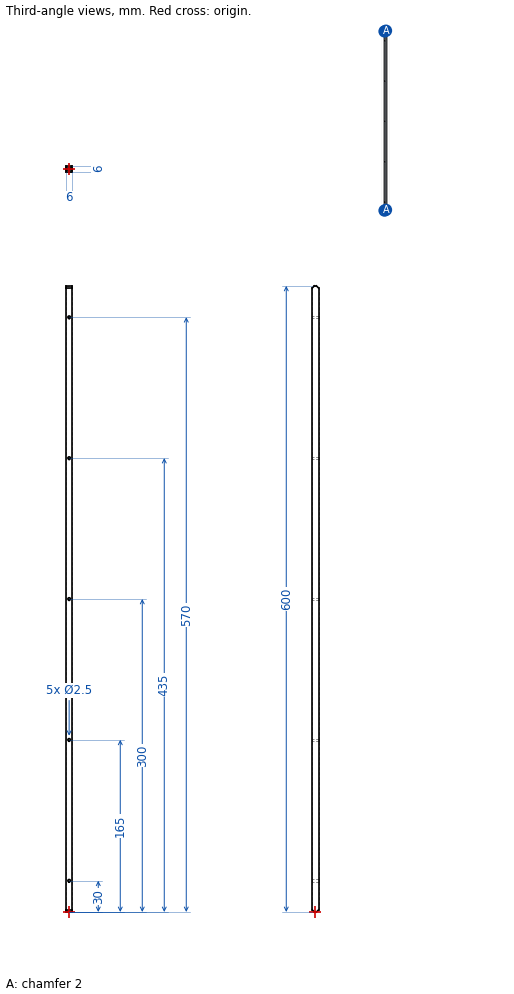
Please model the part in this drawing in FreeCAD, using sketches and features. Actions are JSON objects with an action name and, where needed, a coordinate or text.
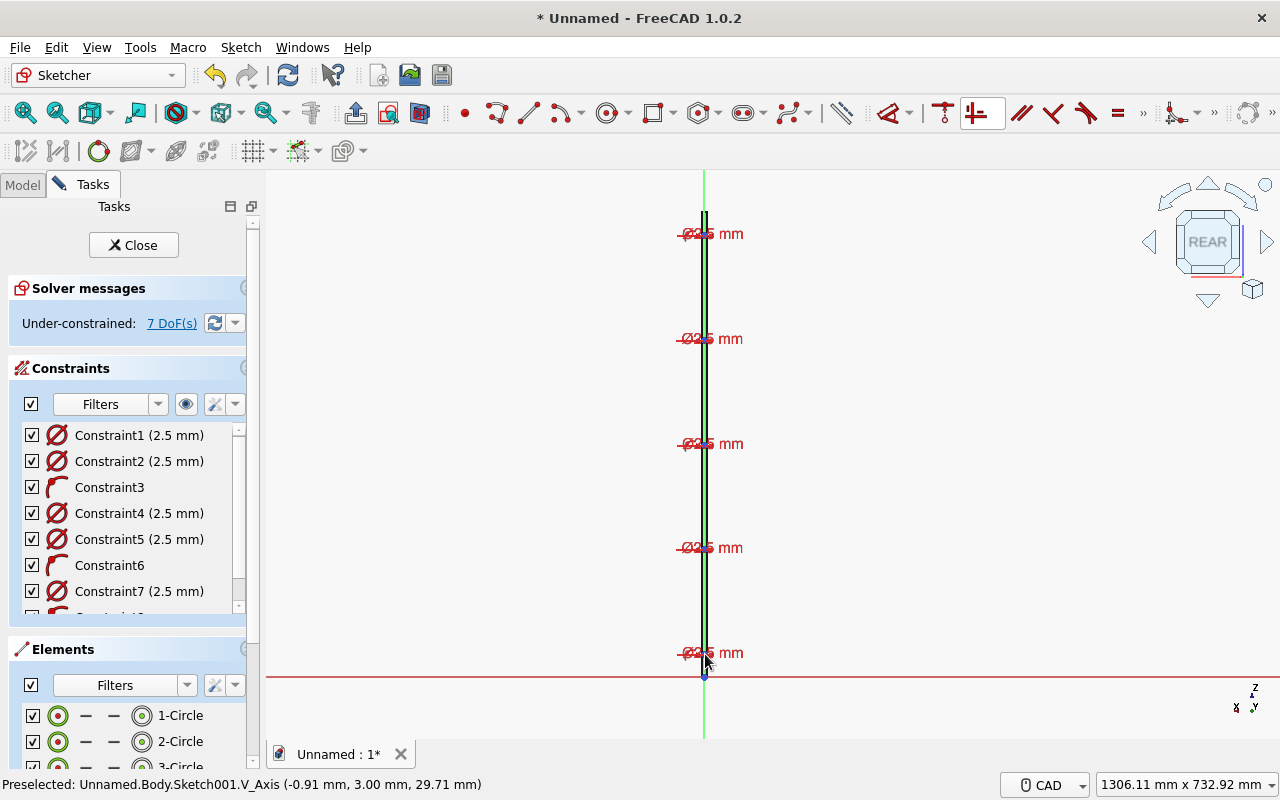
{"action": "left_click", "coordinate": [704, 550]}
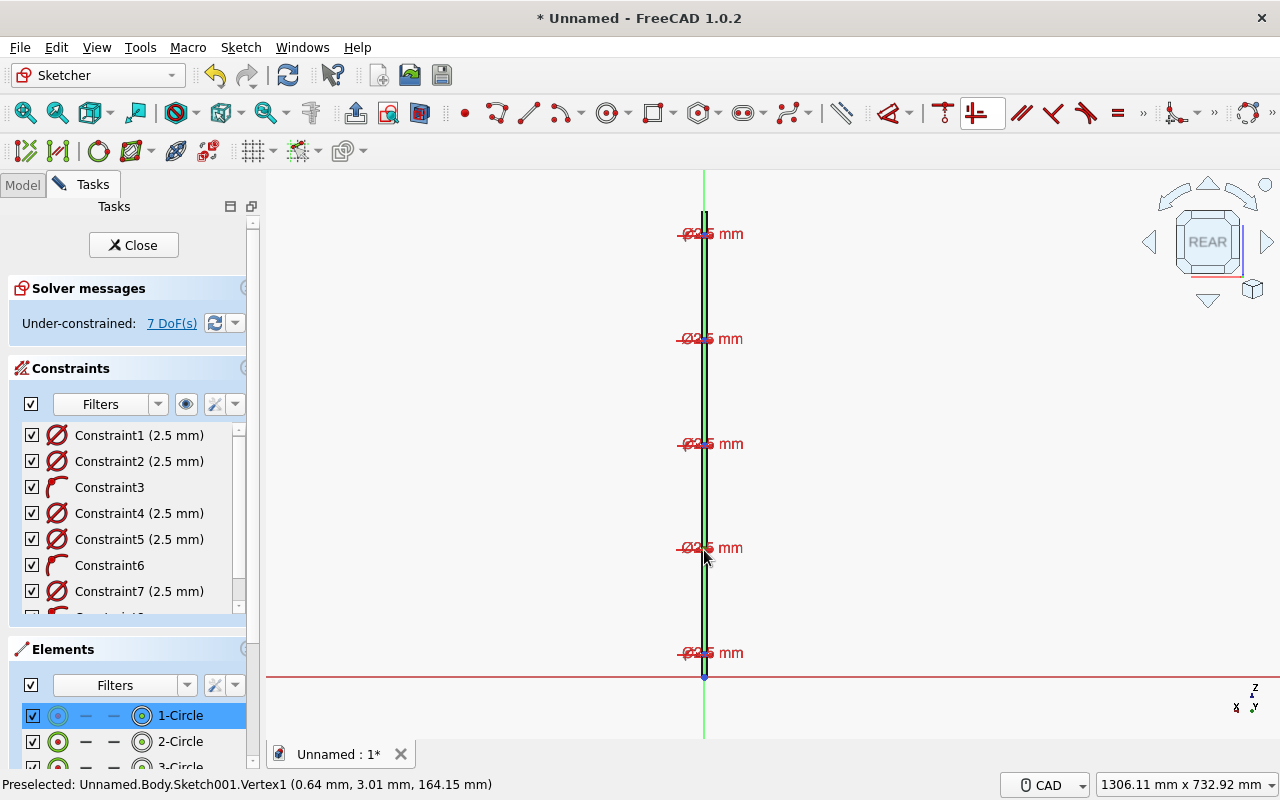
{"action": "left_click", "coordinate": [704, 601]}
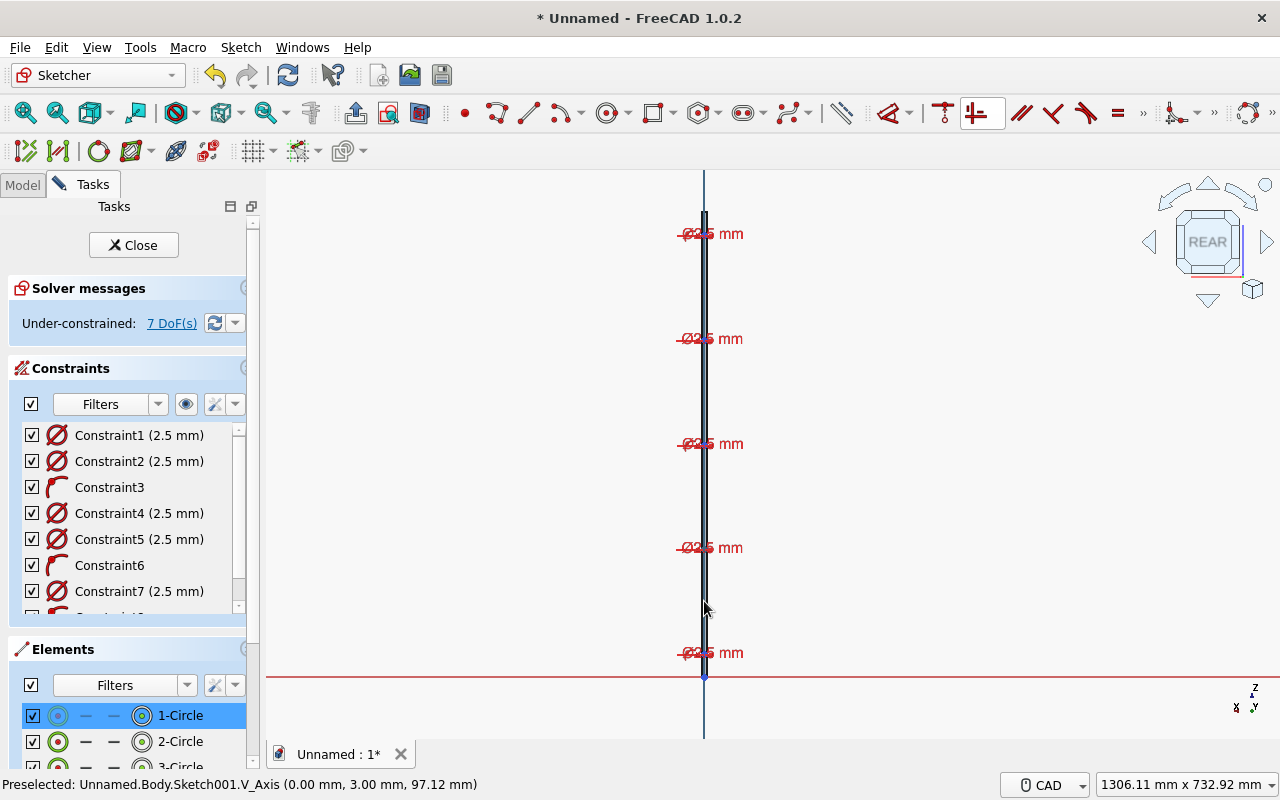
{"action": "left_click", "coordinate": [944, 114]}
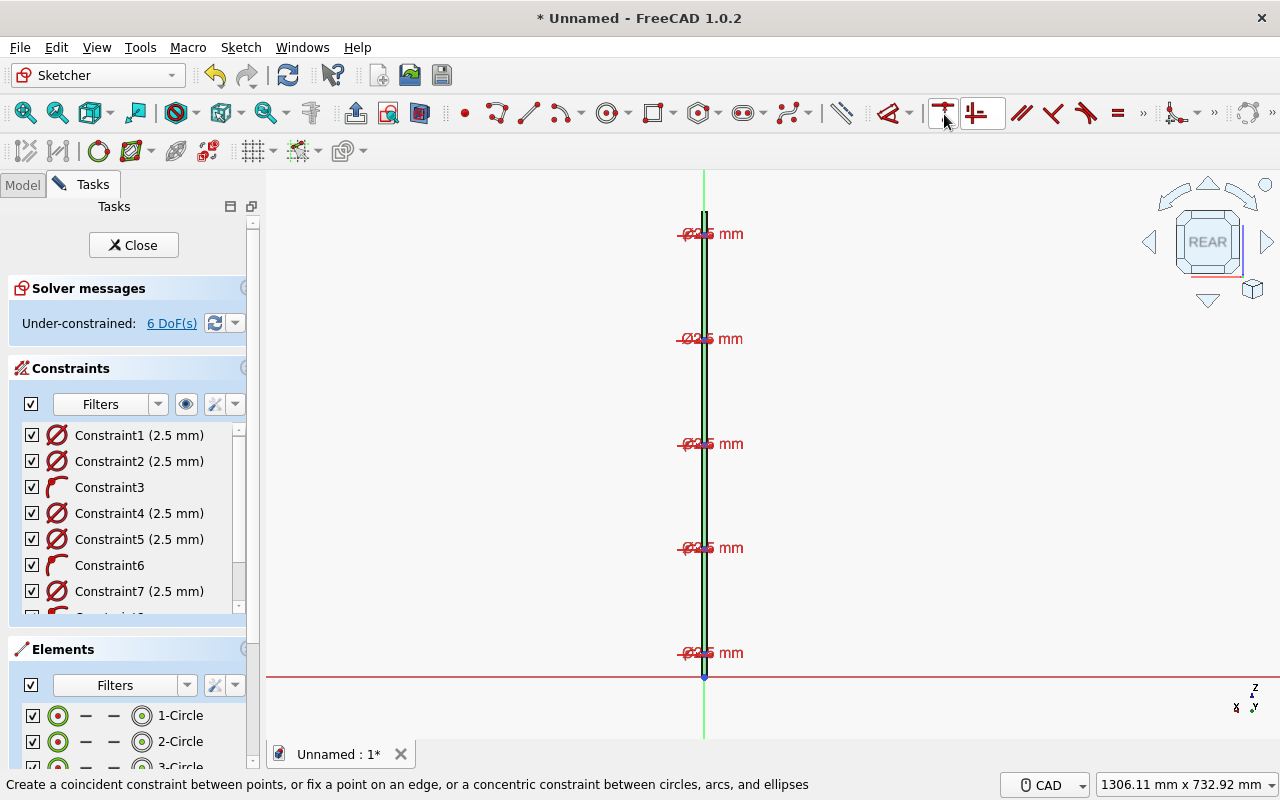
{"action": "left_click", "coordinate": [704, 341]}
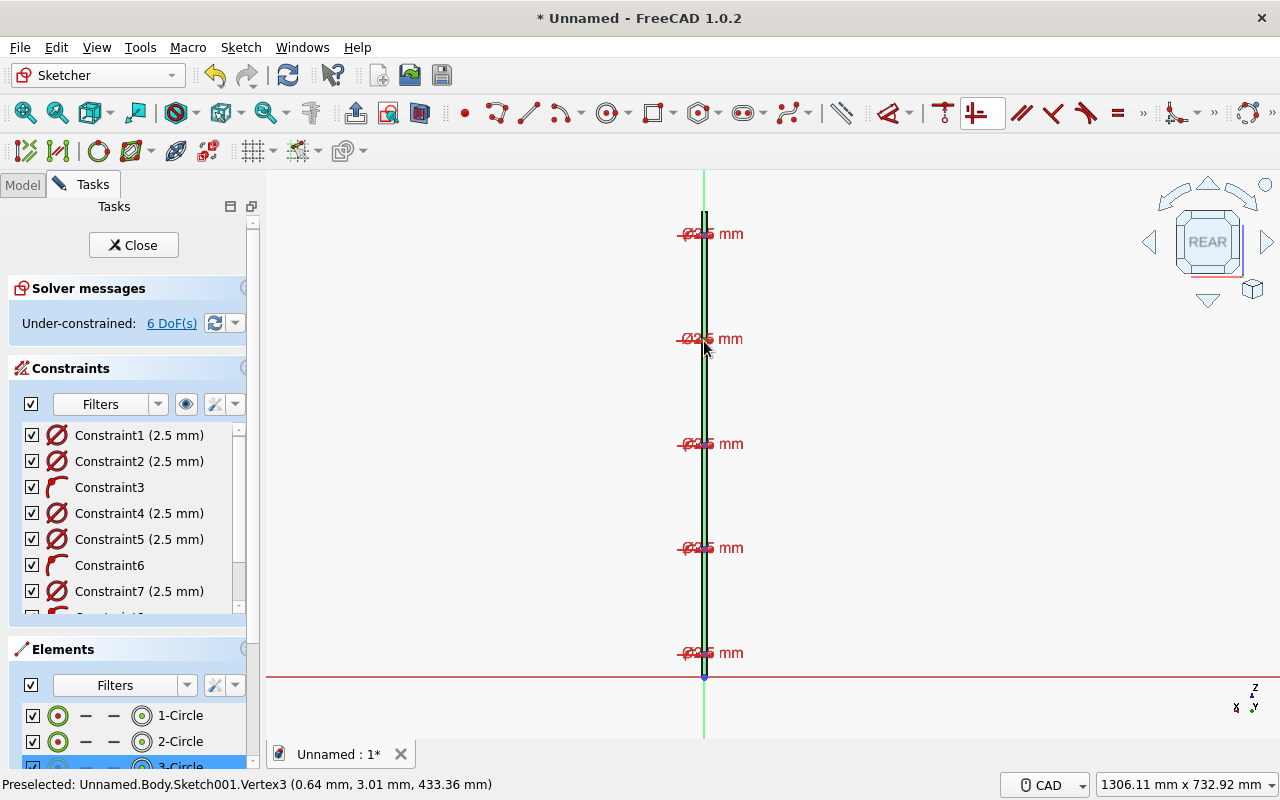
{"action": "left_click", "coordinate": [704, 601]}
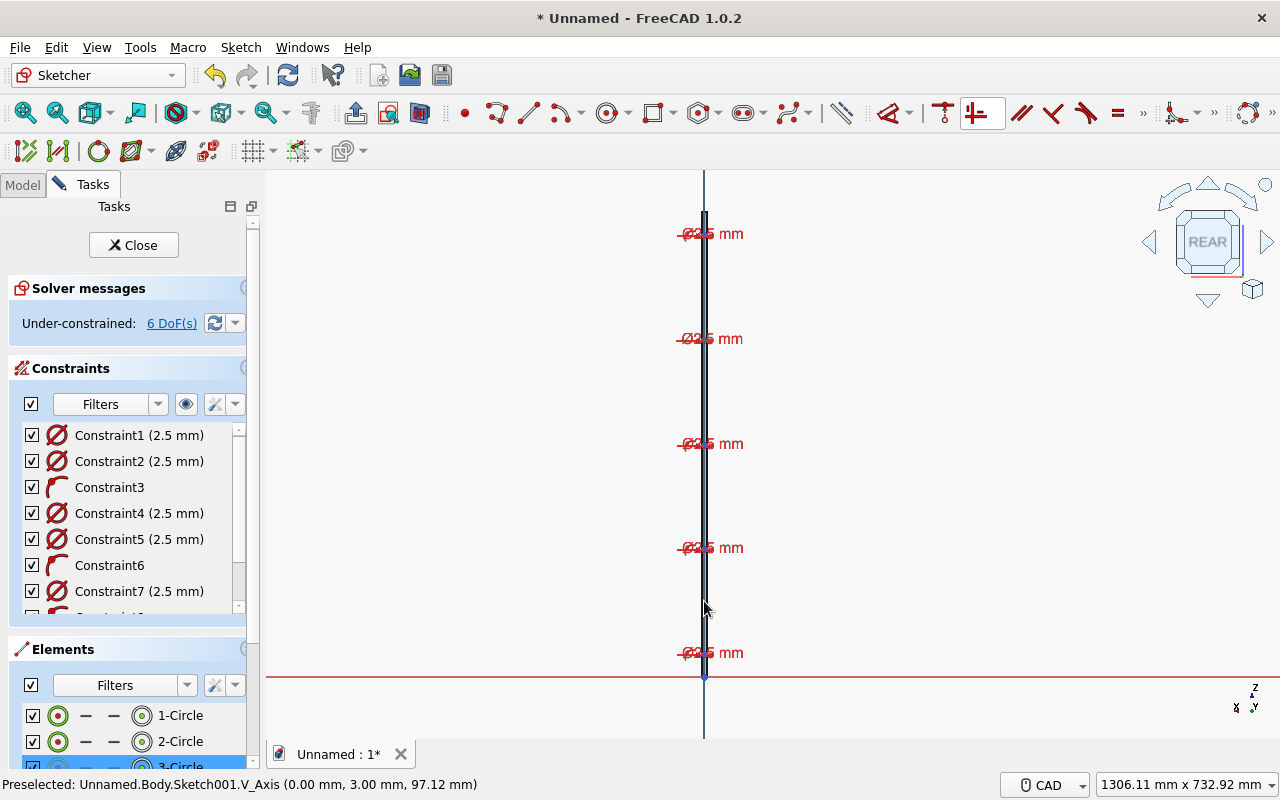
{"action": "left_click", "coordinate": [944, 114]}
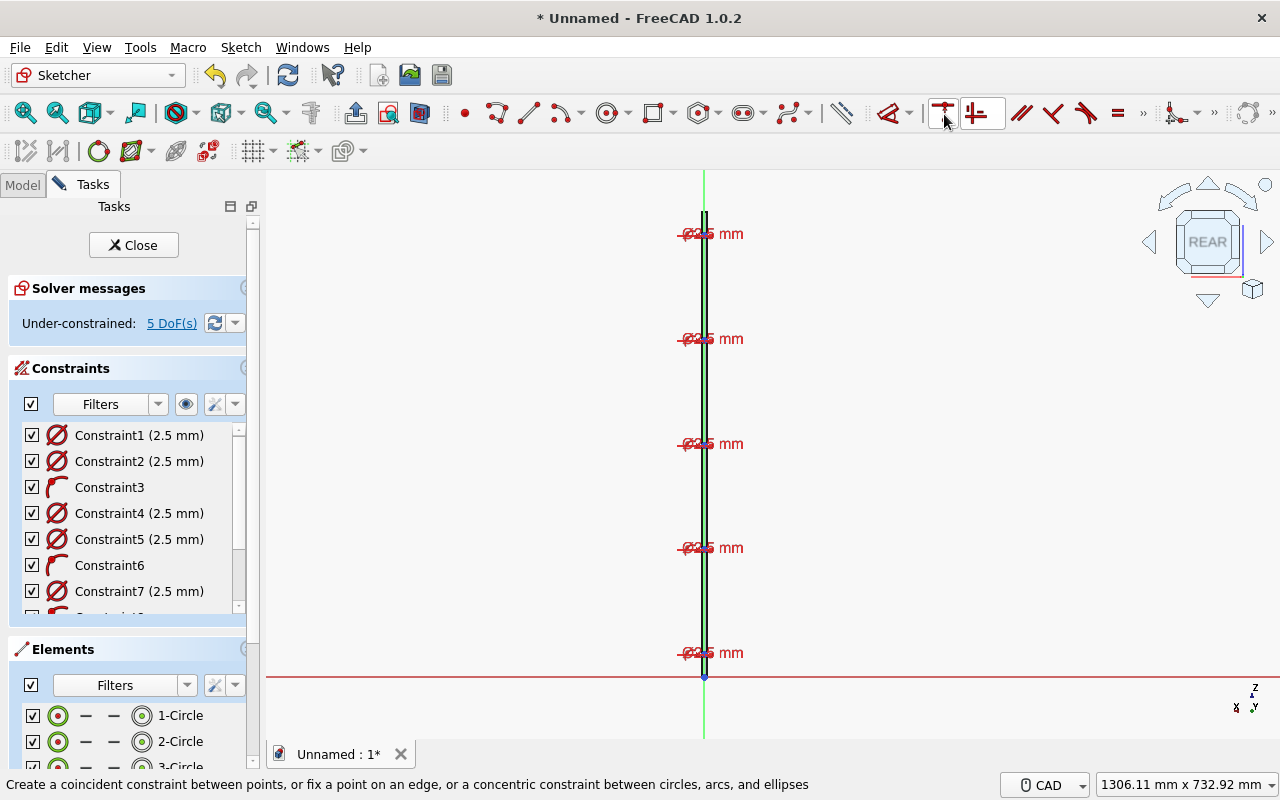
{"action": "left_click", "coordinate": [888, 114]}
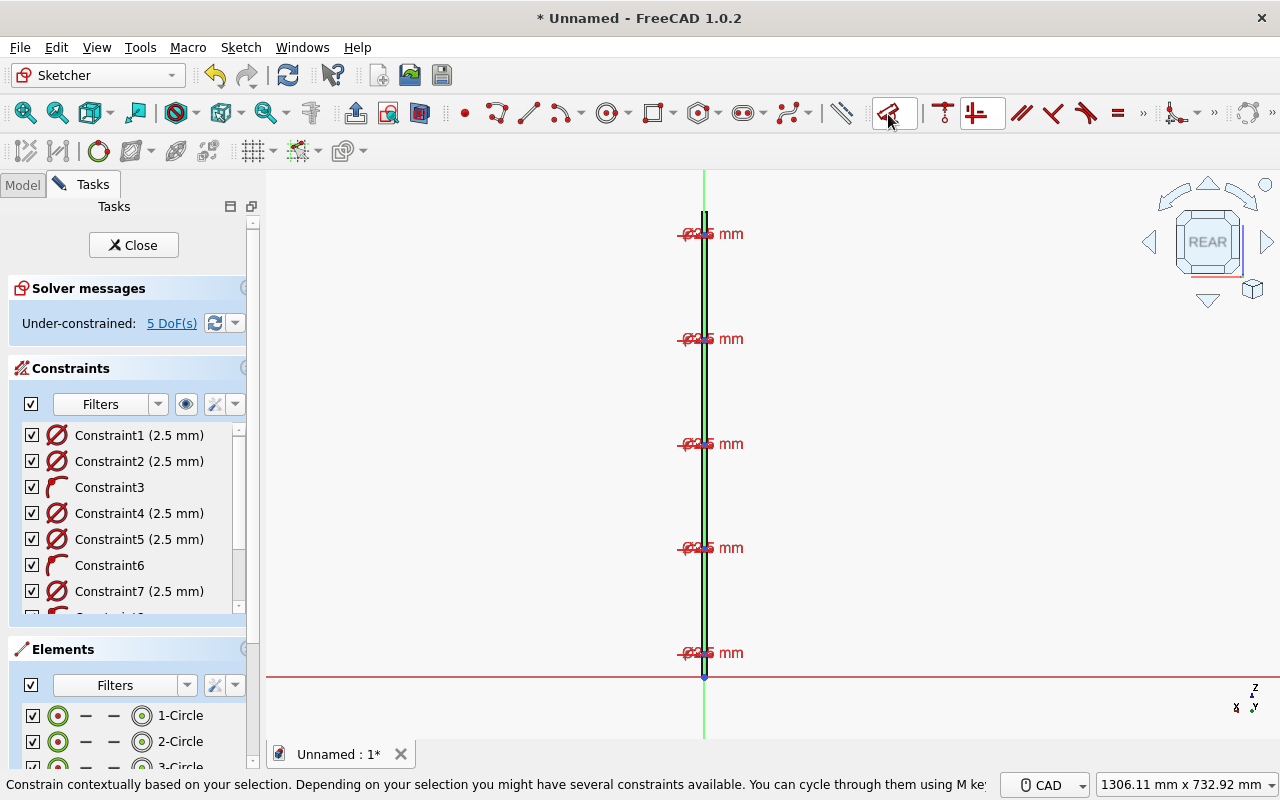
{"action": "scroll", "coordinate": [704, 655], "scroll_direction": "up", "scroll_amount": 3}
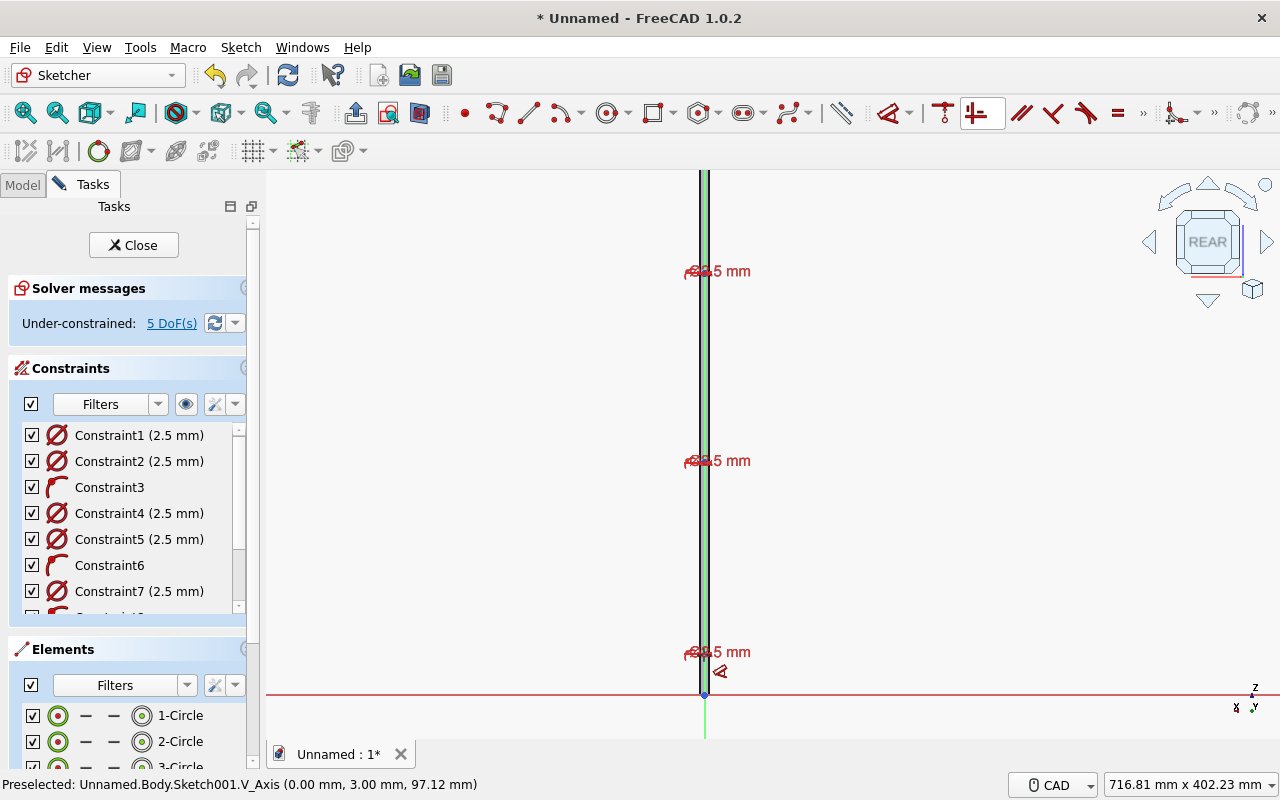
{"action": "left_click", "coordinate": [705, 654]}
{"action": "left_click", "coordinate": [739, 675]}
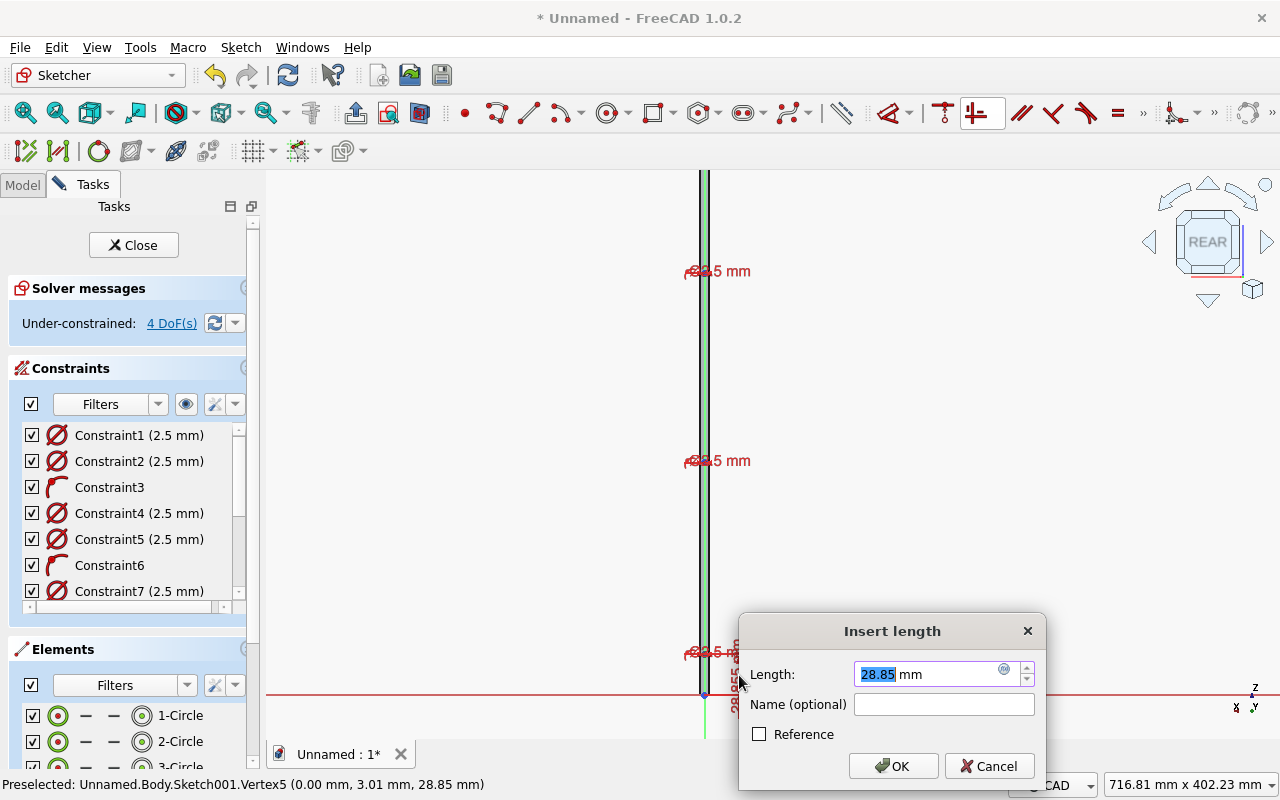
{"action": "type", "text": "30"}
{"action": "key", "text": "Return"}